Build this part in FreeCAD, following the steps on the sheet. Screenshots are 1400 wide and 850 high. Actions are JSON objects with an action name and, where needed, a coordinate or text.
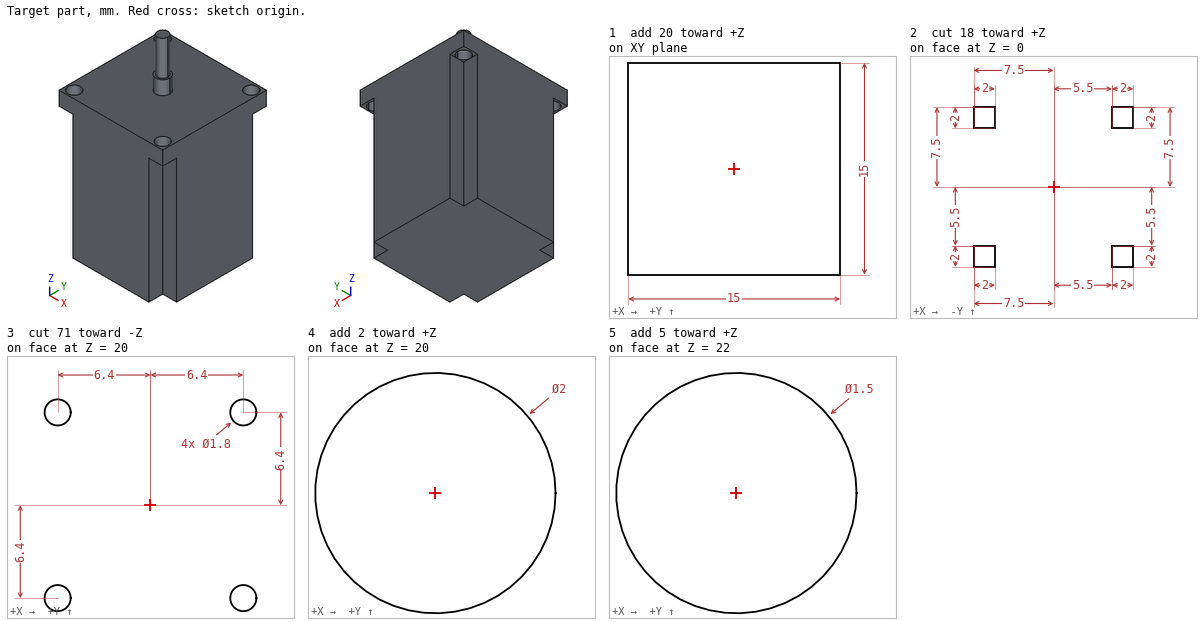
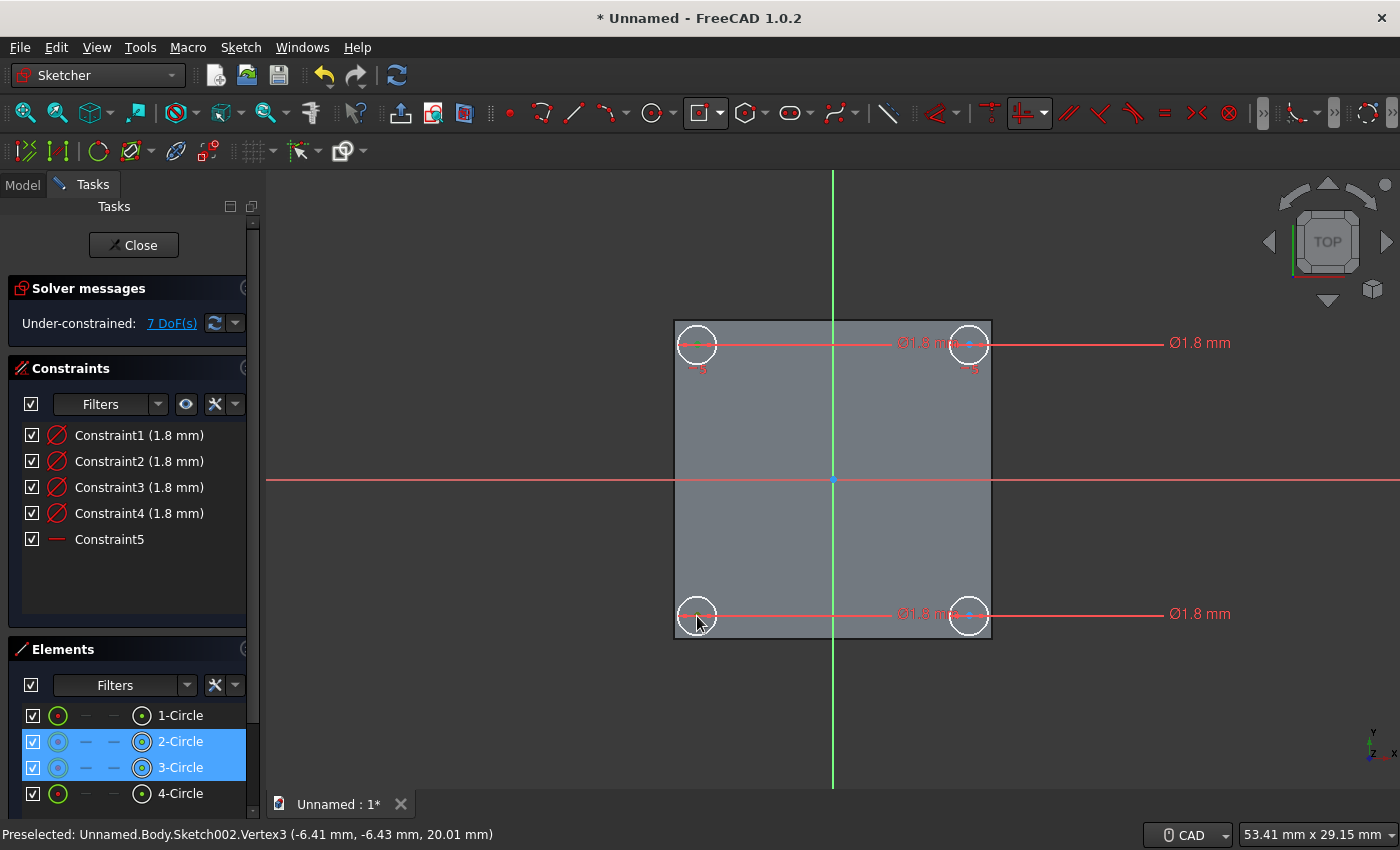
{"action": "key", "text": "v"}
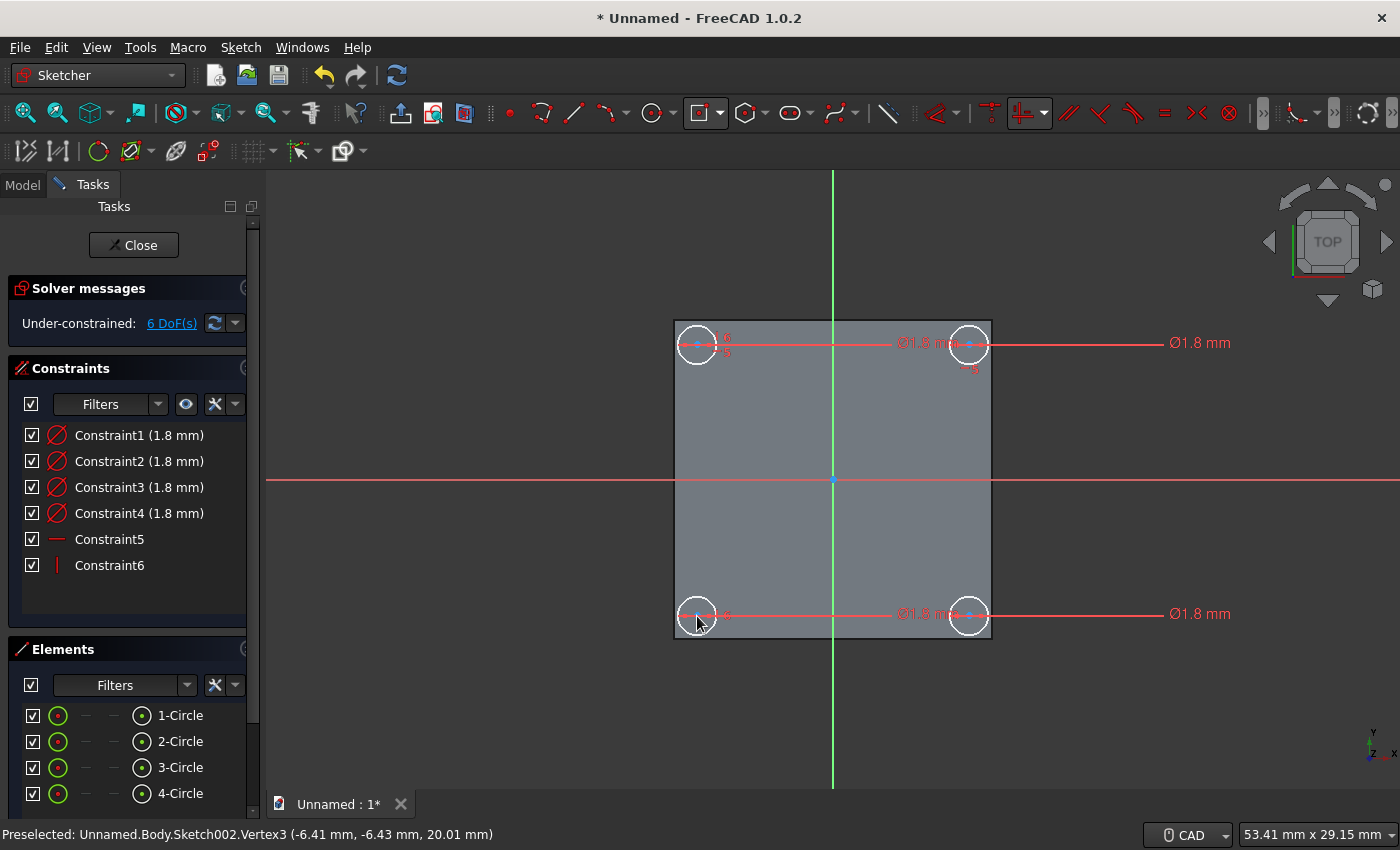
{"action": "left_click", "coordinate": [969, 345]}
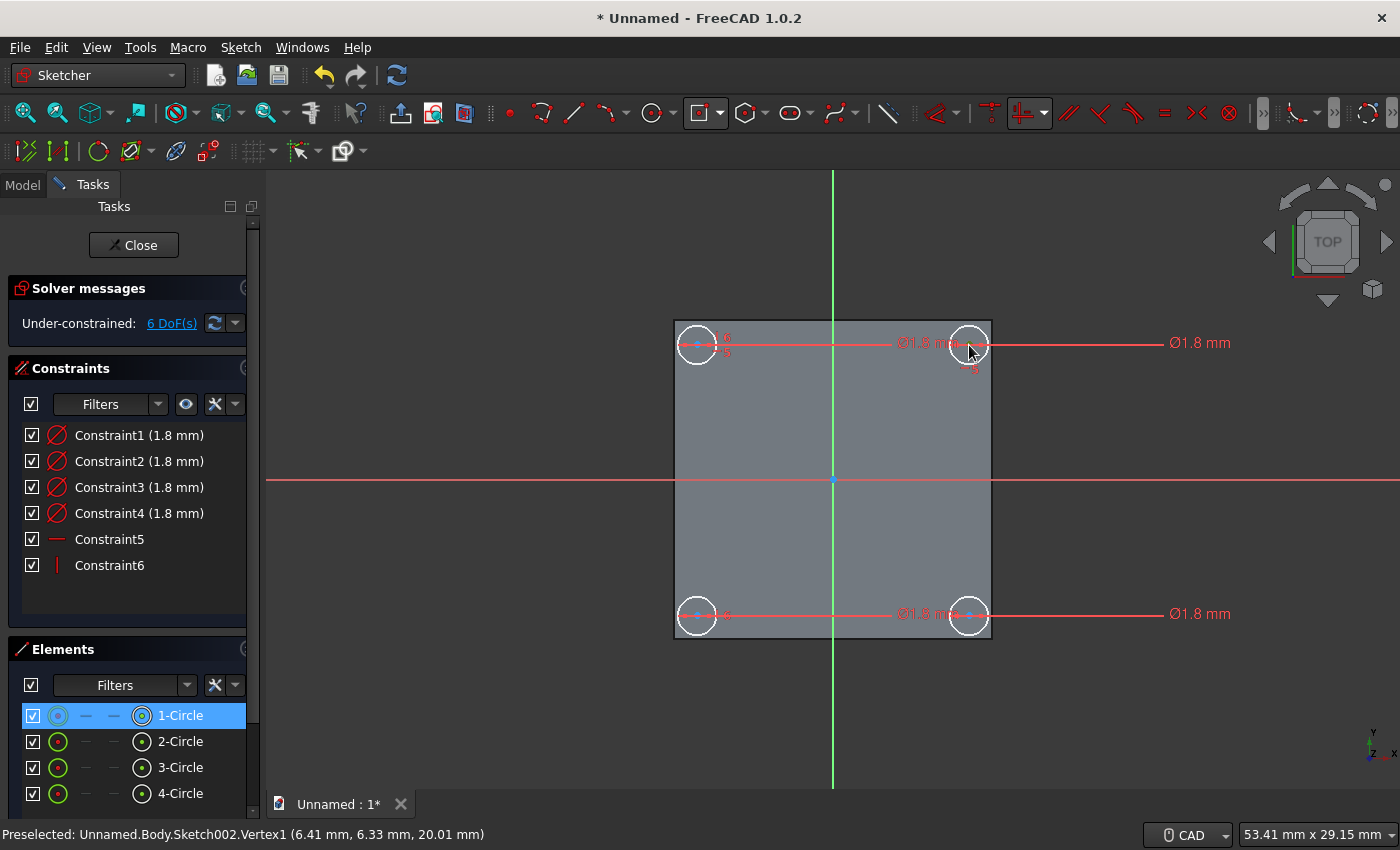
{"action": "left_click", "coordinate": [969, 616]}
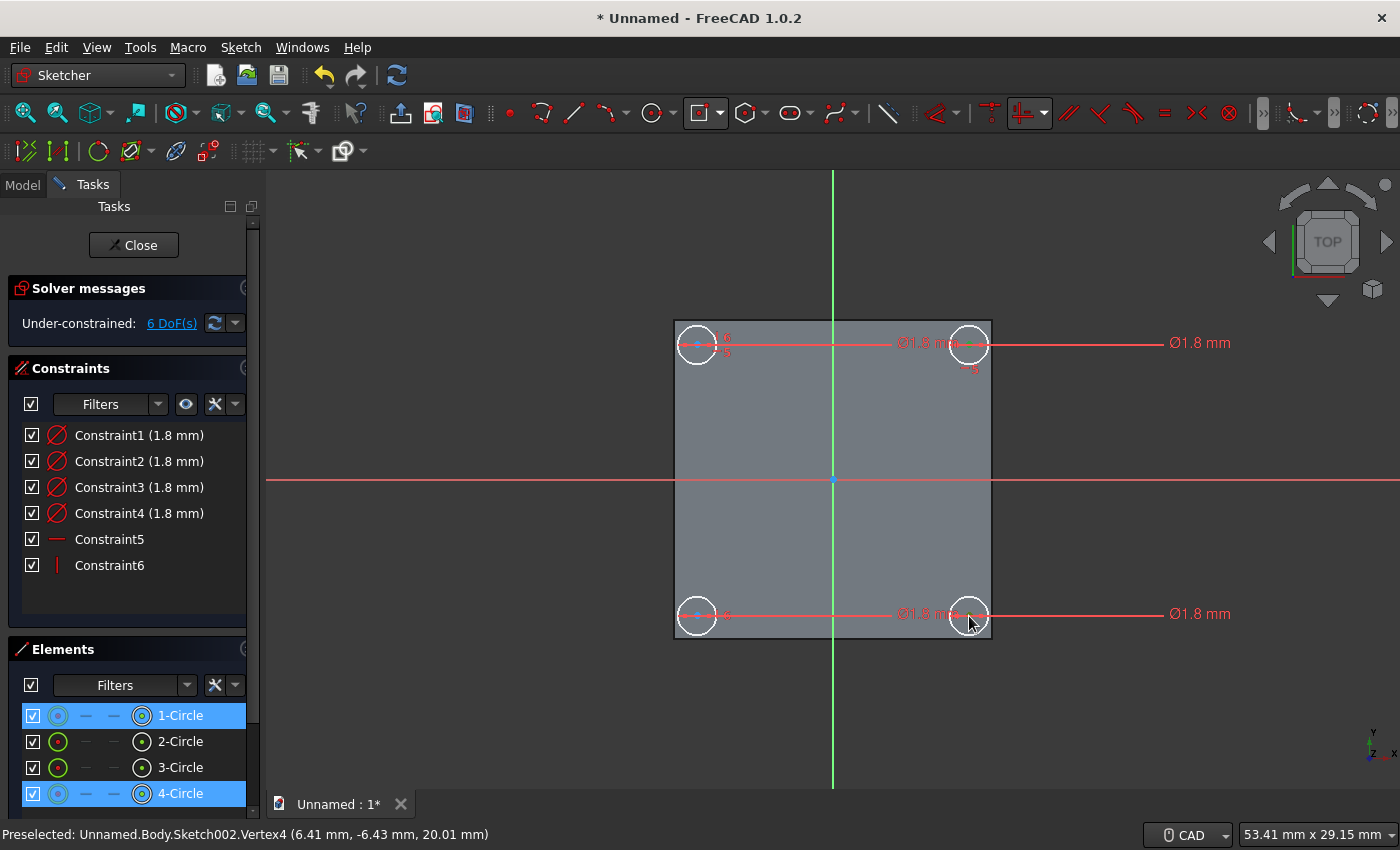
{"action": "key", "text": "v"}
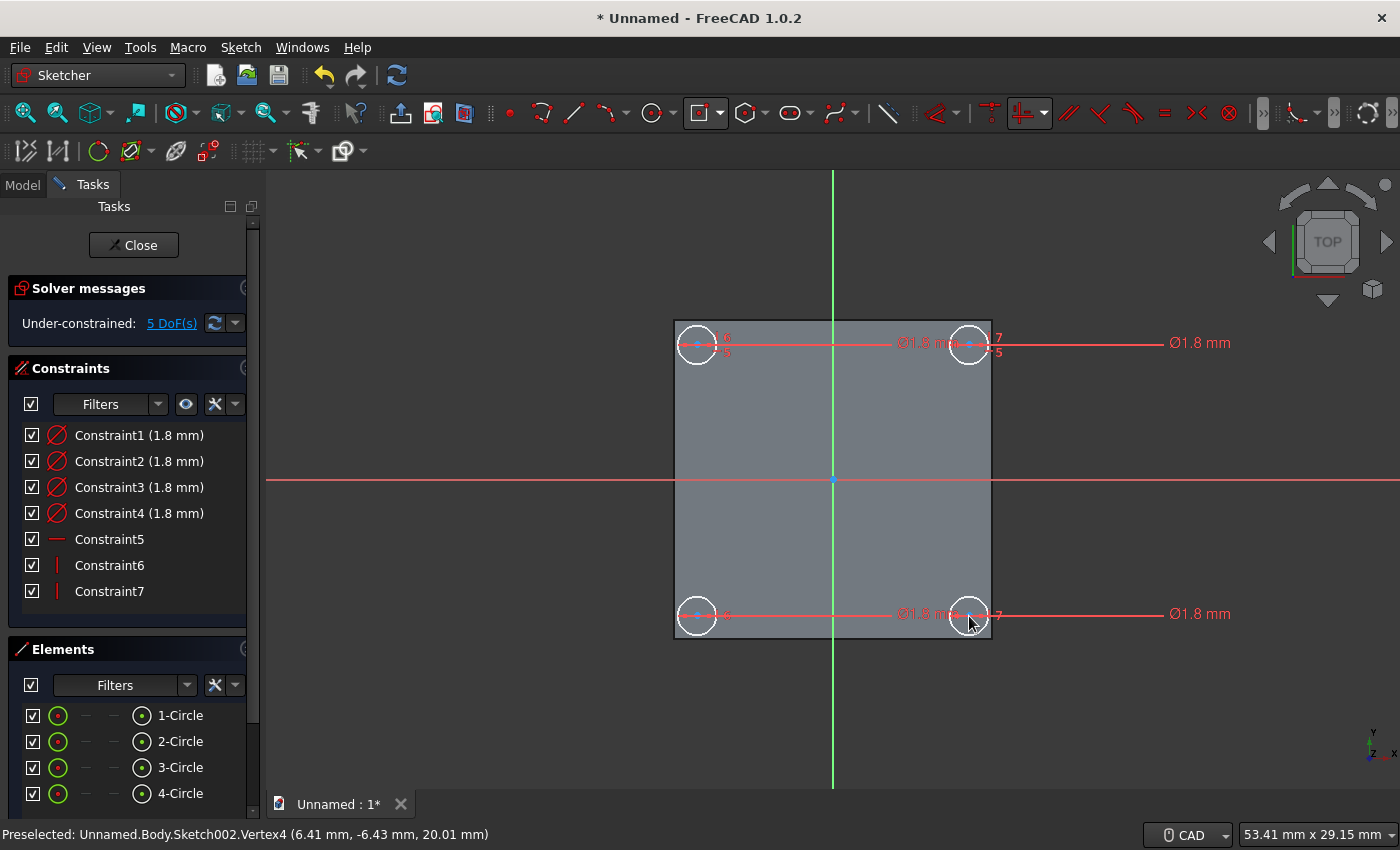
{"action": "left_click", "coordinate": [697, 616]}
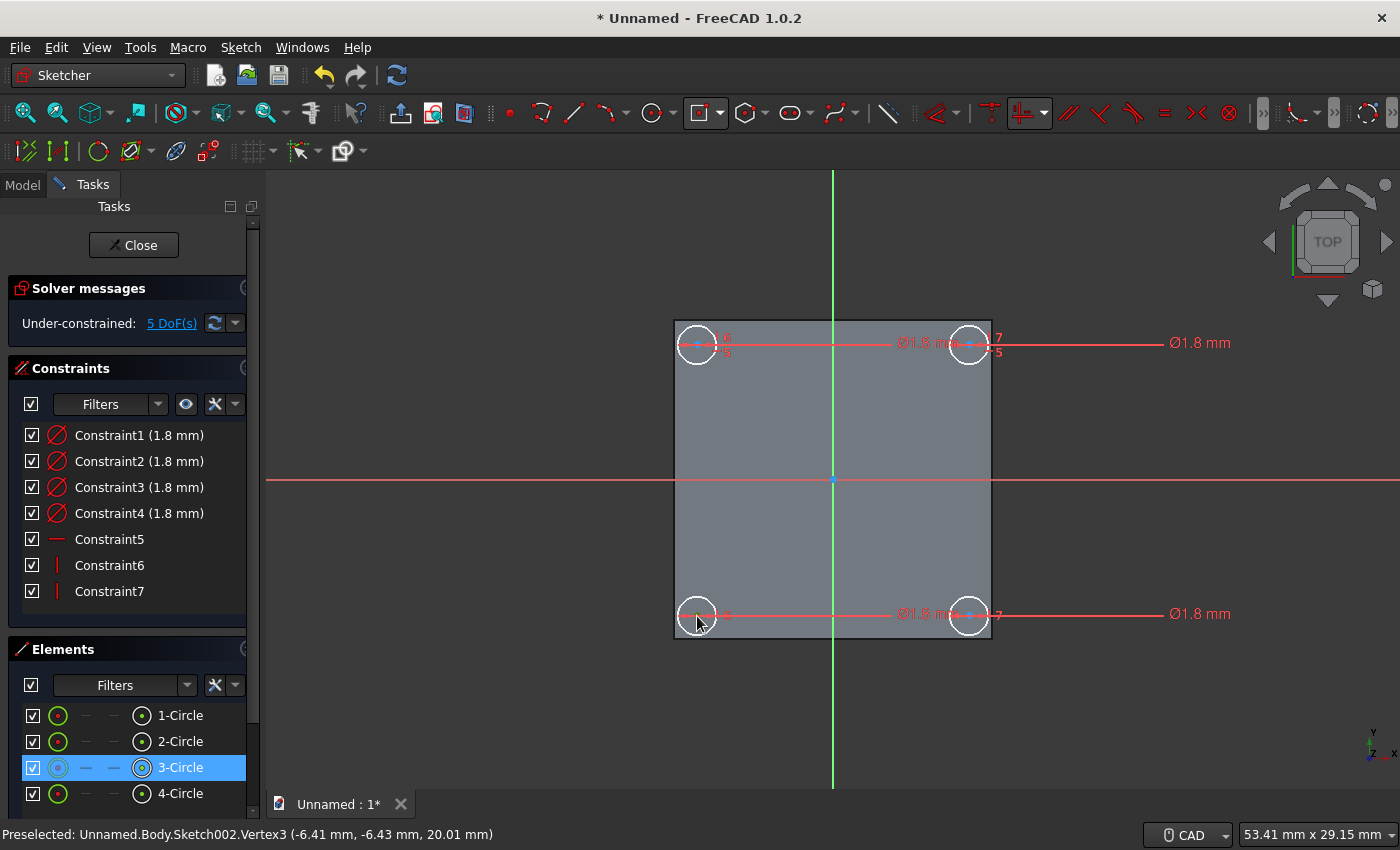
{"action": "left_click", "coordinate": [969, 616]}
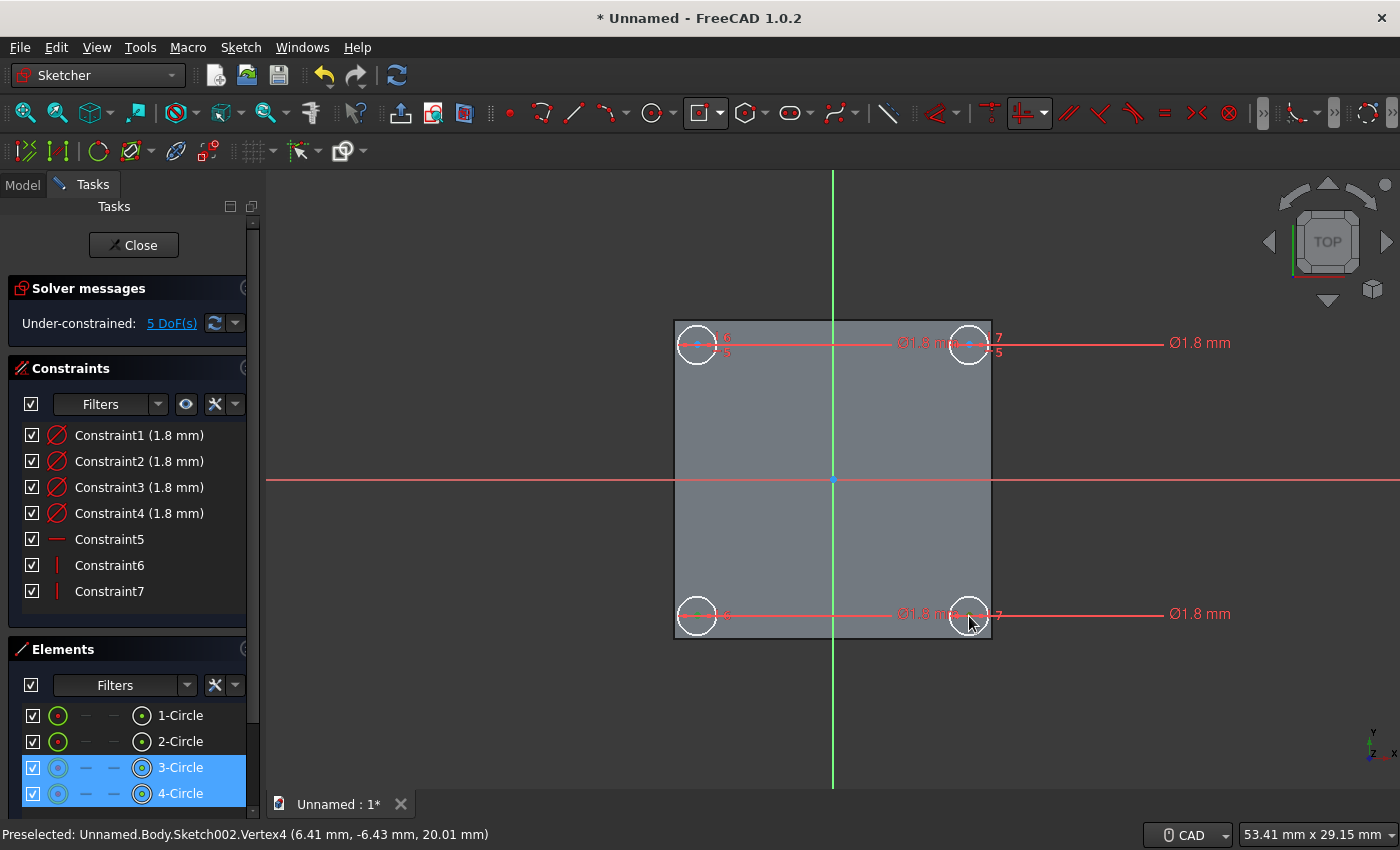
{"action": "key", "text": "h"}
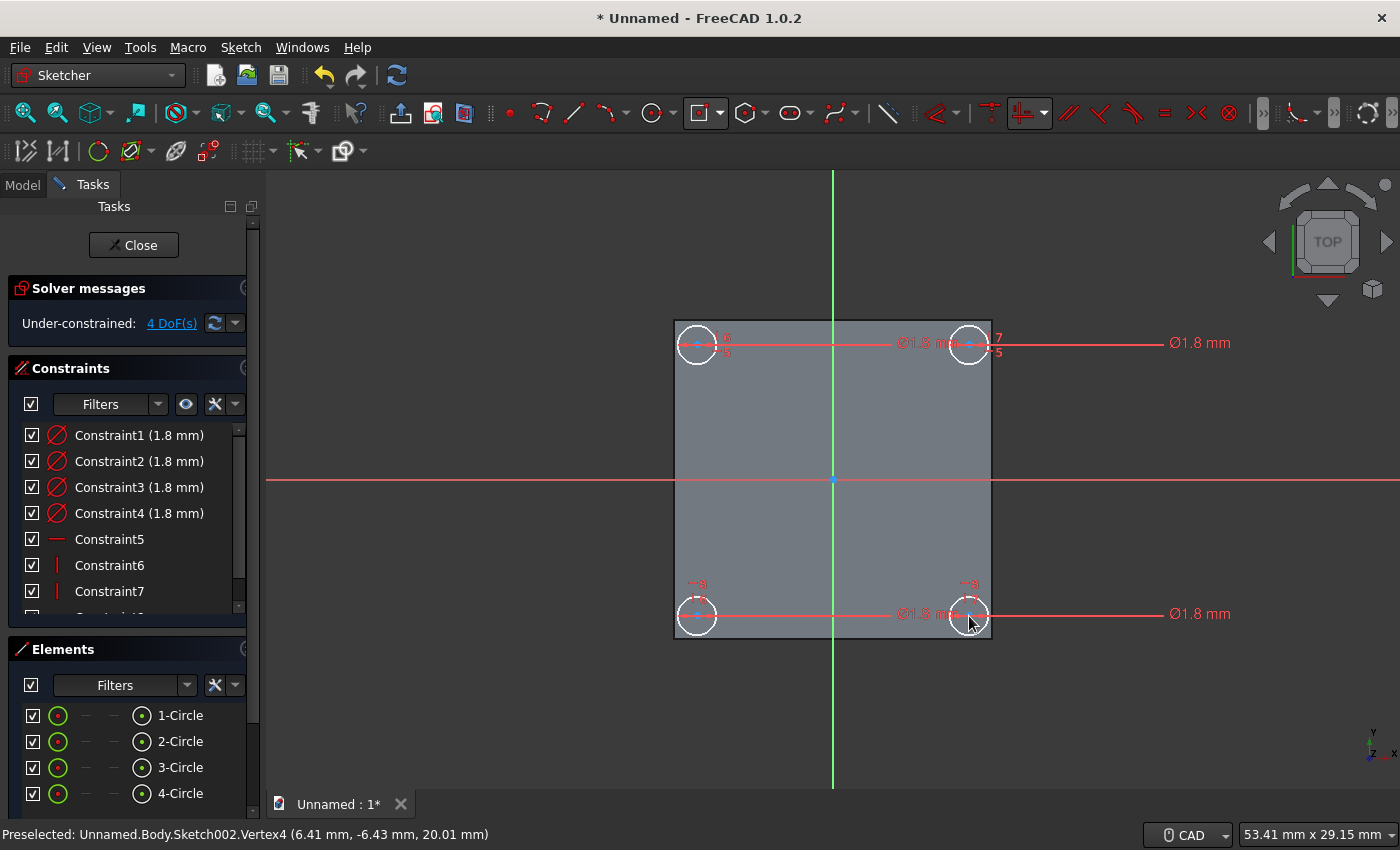
{"action": "left_click", "coordinate": [936, 114]}